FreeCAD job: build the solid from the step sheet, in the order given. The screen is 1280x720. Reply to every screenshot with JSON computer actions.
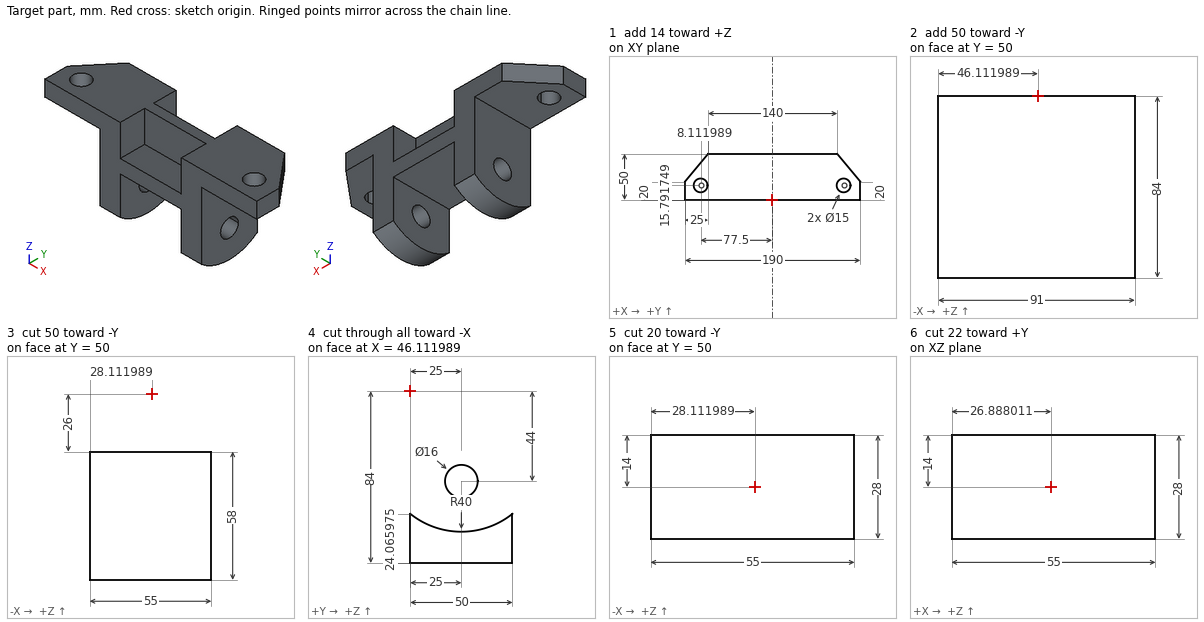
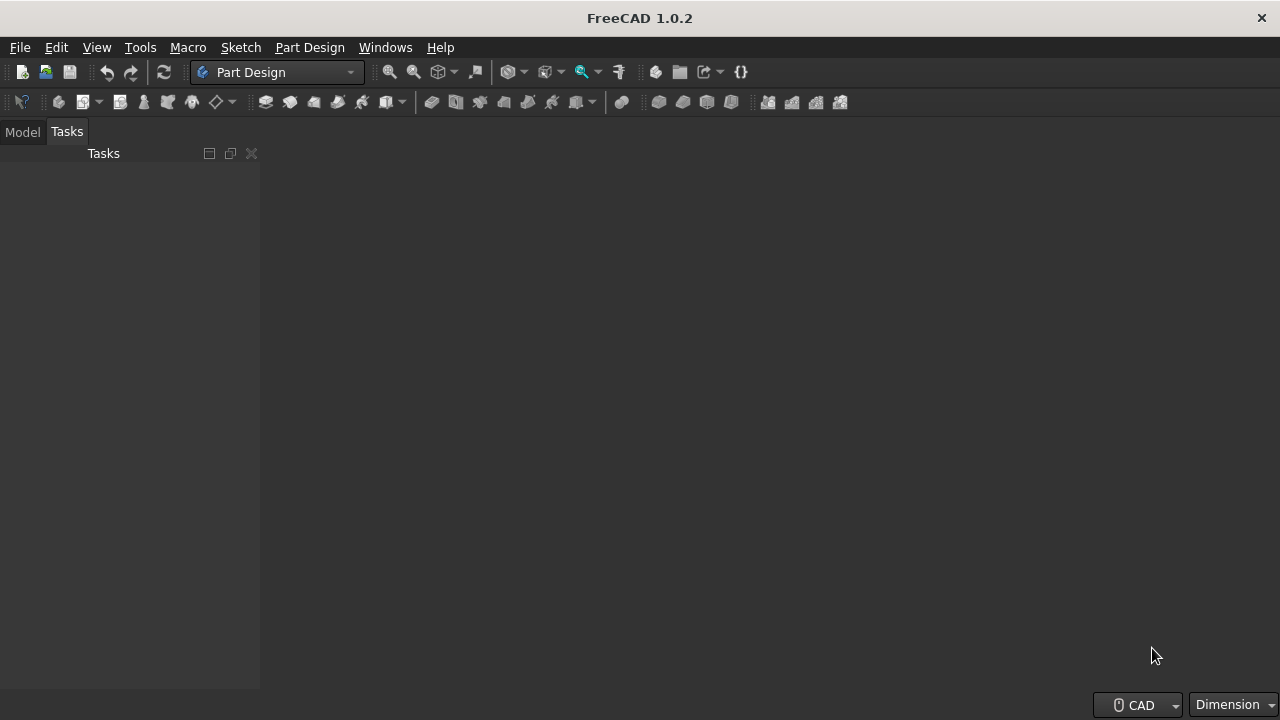
{"action": "left_click", "coordinate": [22, 72]}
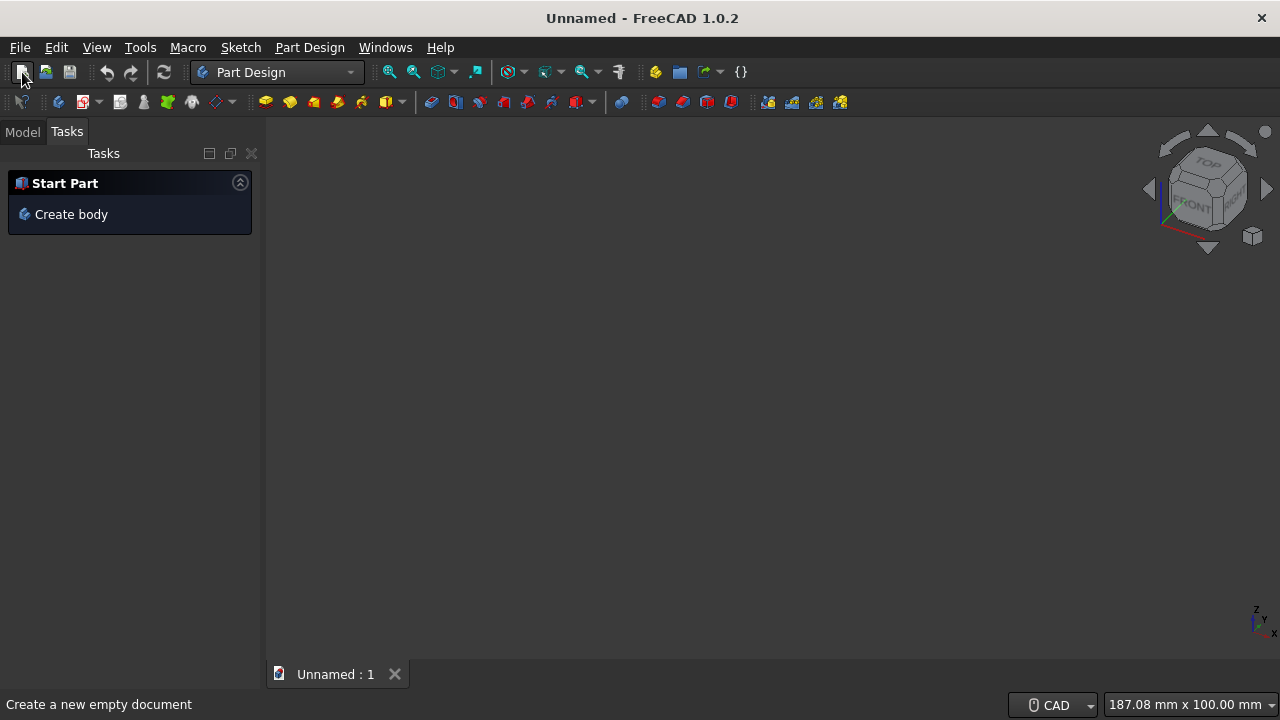
{"action": "left_click", "coordinate": [84, 102]}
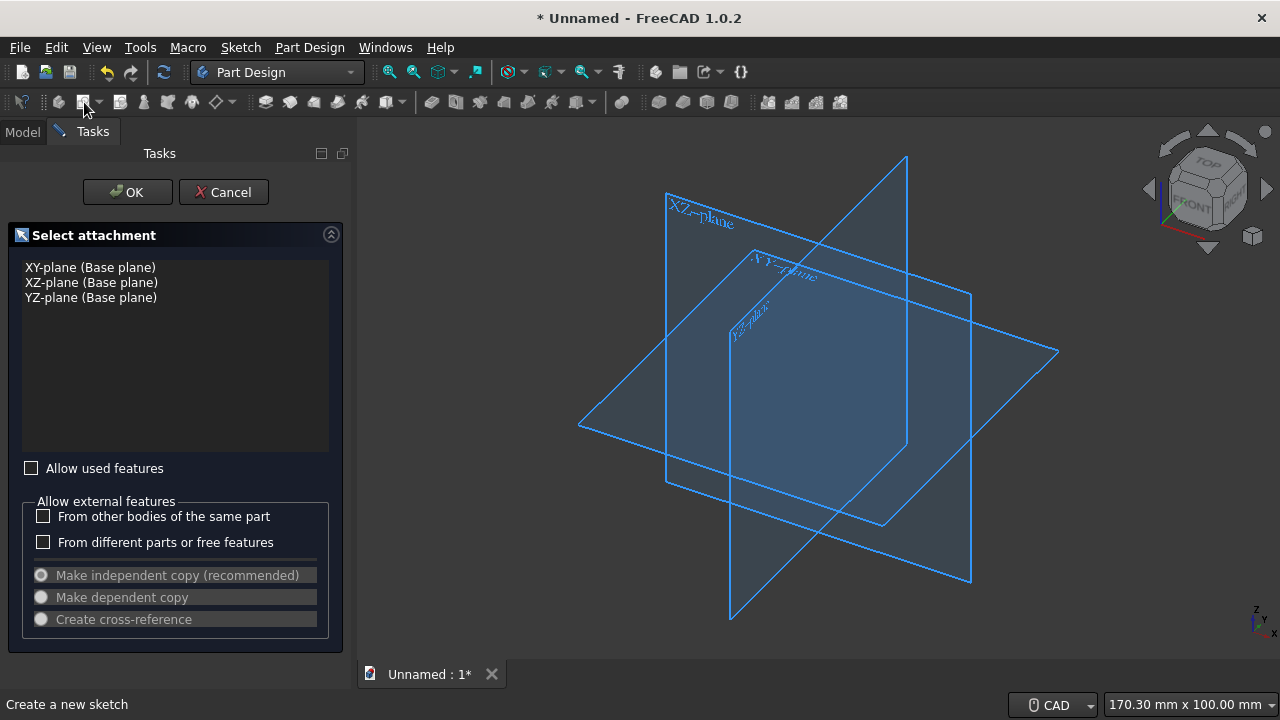
{"action": "left_click", "coordinate": [82, 268]}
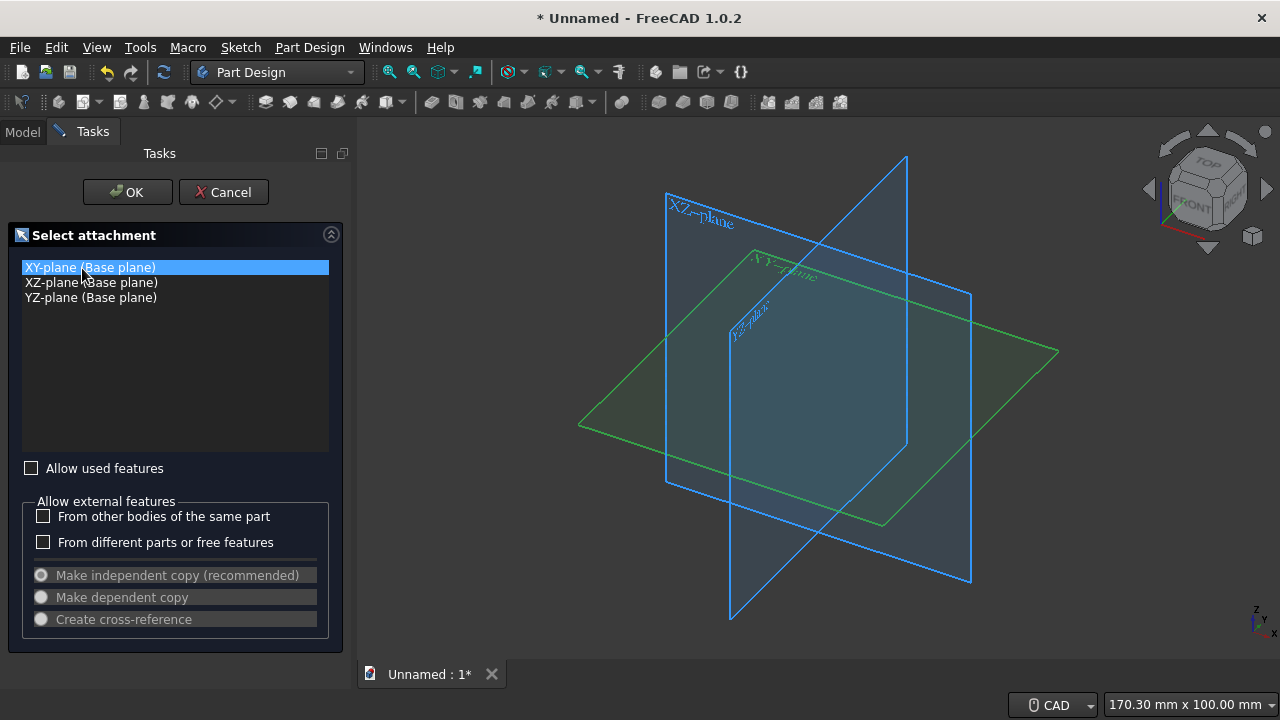
{"action": "left_click", "coordinate": [128, 192]}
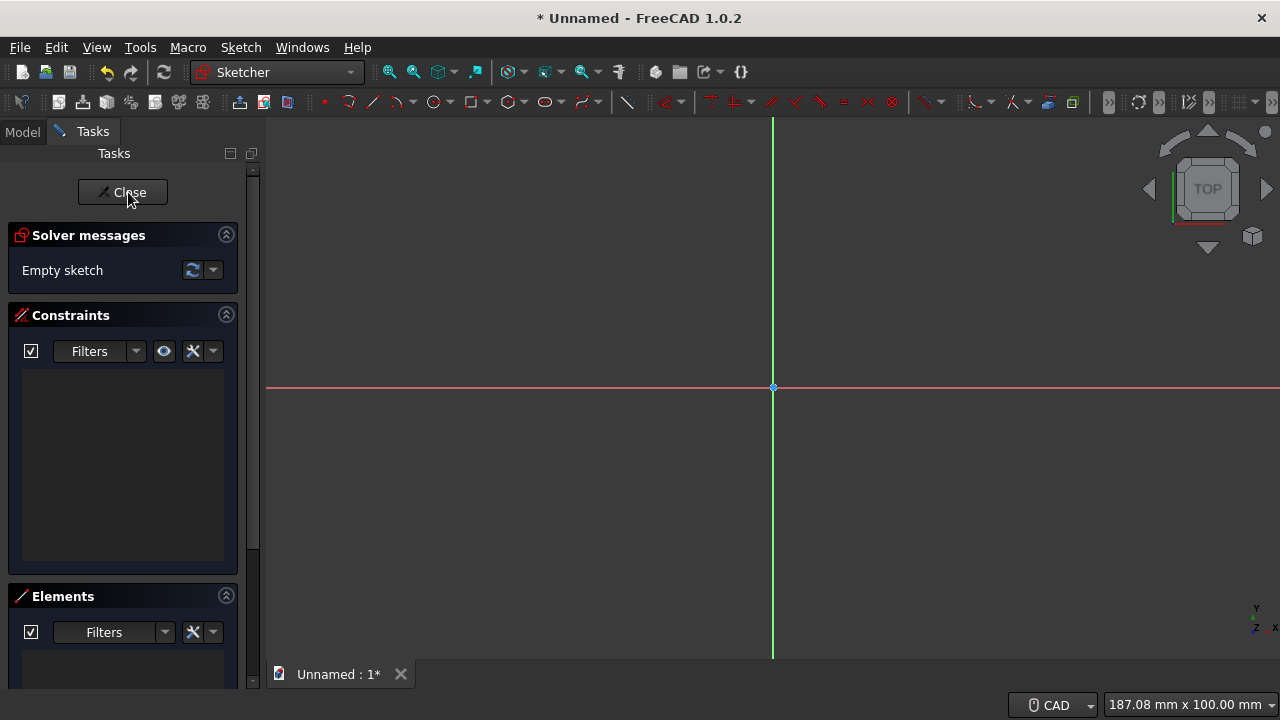
{"action": "scroll", "coordinate": [617, 553], "scroll_direction": "down", "scroll_amount": 3}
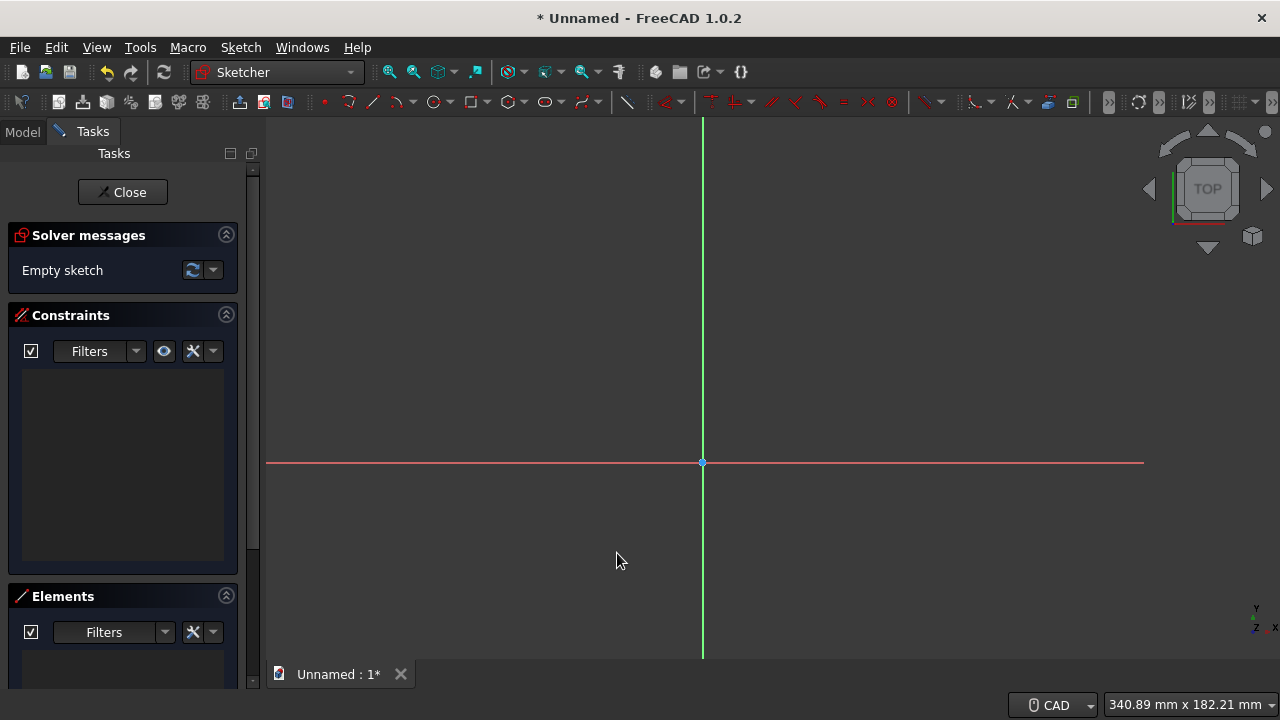
{"action": "left_click", "coordinate": [350, 102]}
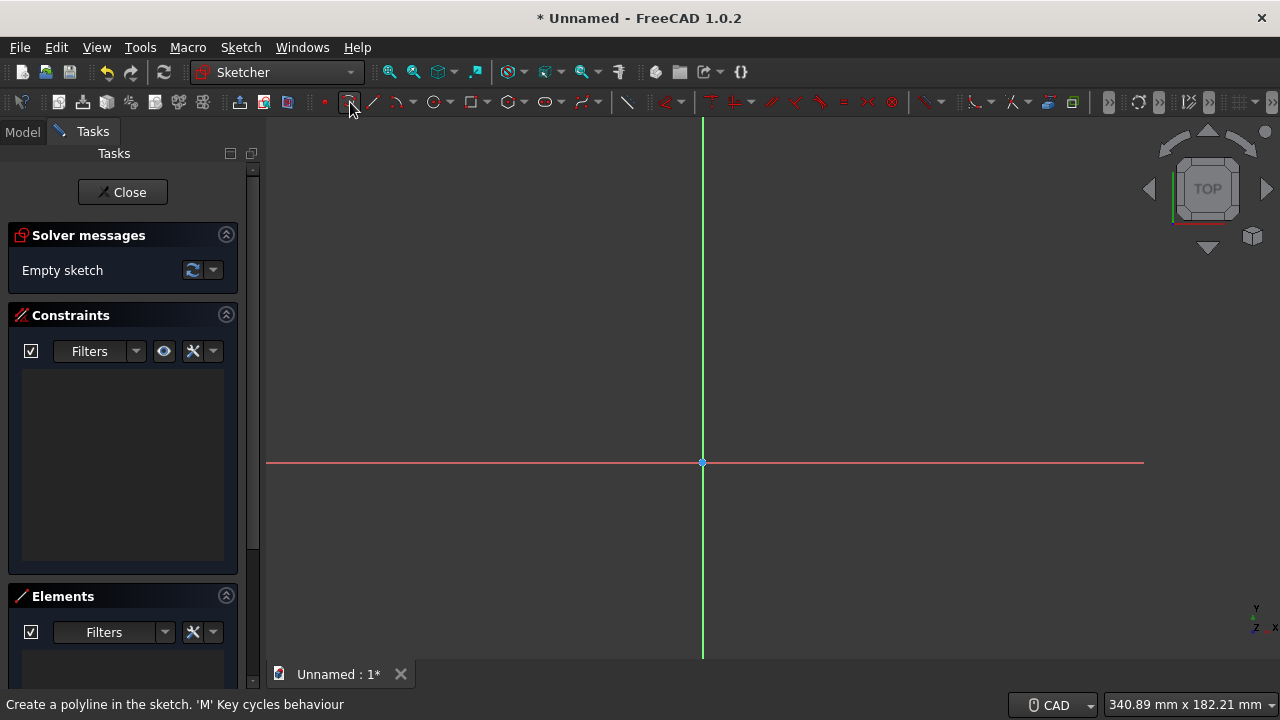
{"action": "left_click", "coordinate": [496, 314]}
{"action": "left_click", "coordinate": [422, 403]}
{"action": "left_click", "coordinate": [422, 463]}
{"action": "left_click", "coordinate": [987, 454]}
{"action": "left_click", "coordinate": [987, 403]}
{"action": "left_click", "coordinate": [913, 314]}
{"action": "left_click", "coordinate": [496, 315]}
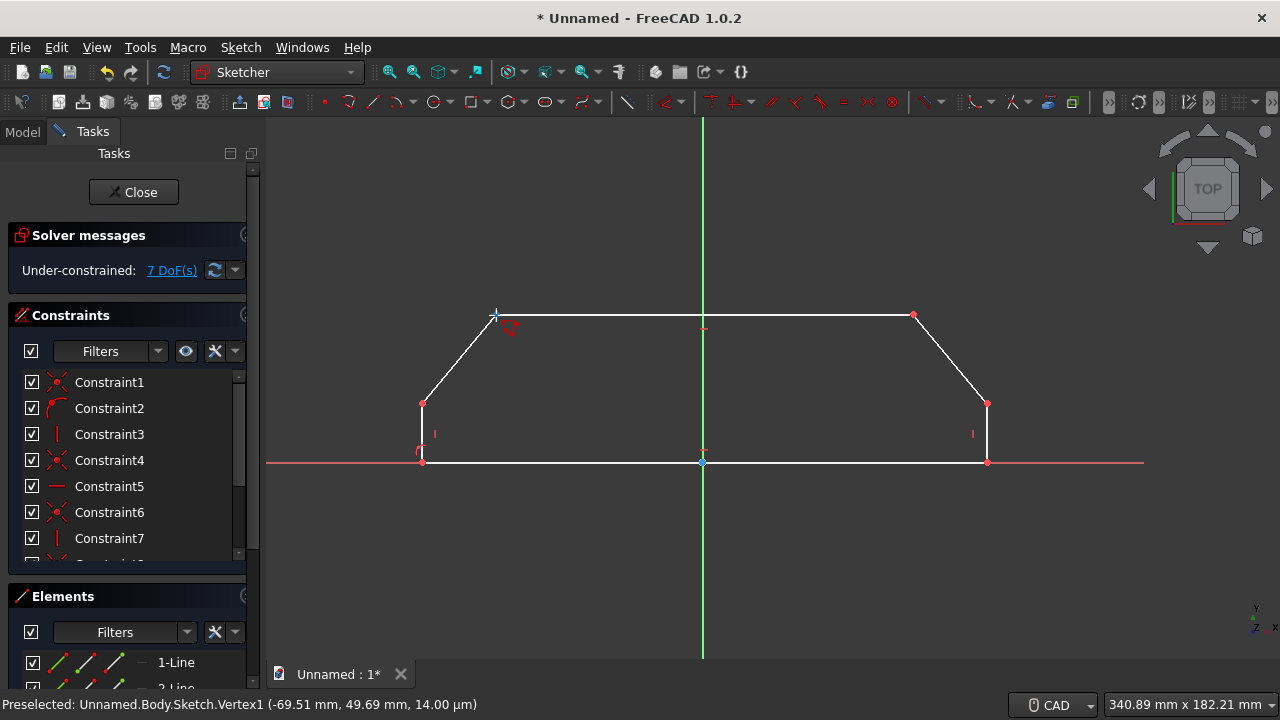
{"action": "left_click", "coordinate": [434, 102]}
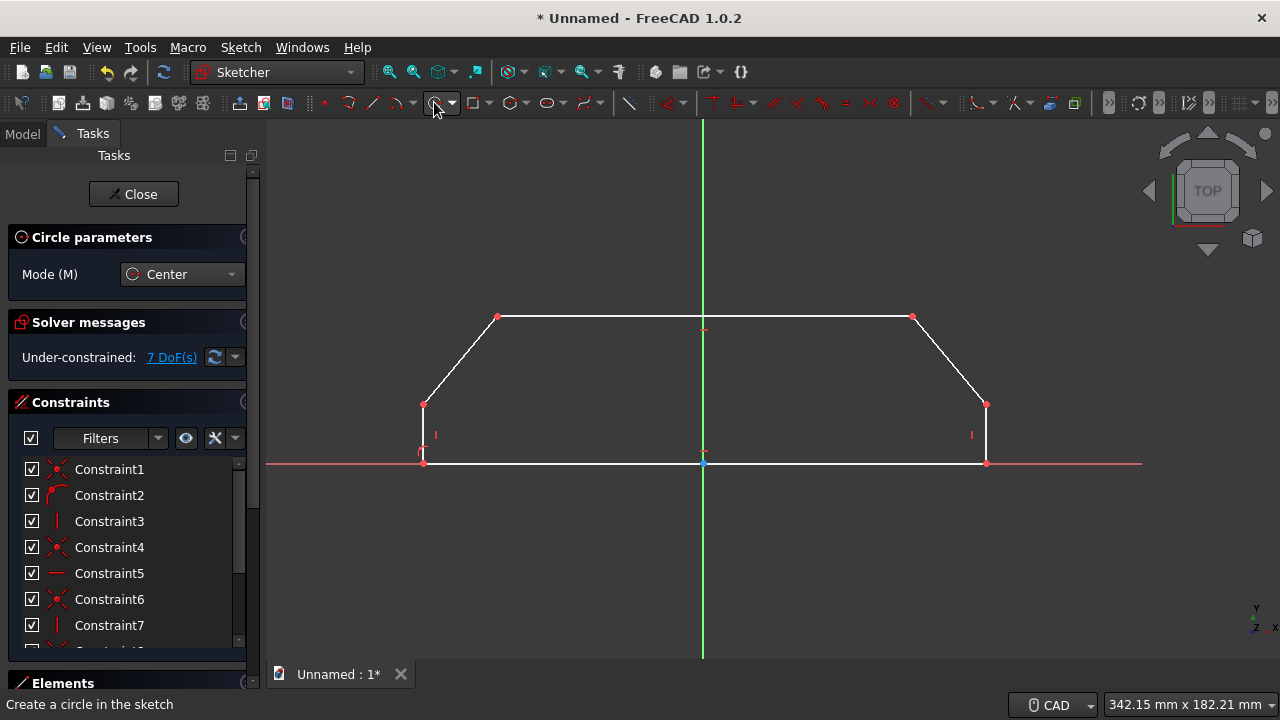
{"action": "left_click", "coordinate": [473, 417]}
{"action": "mouse_move", "coordinate": [489, 401]}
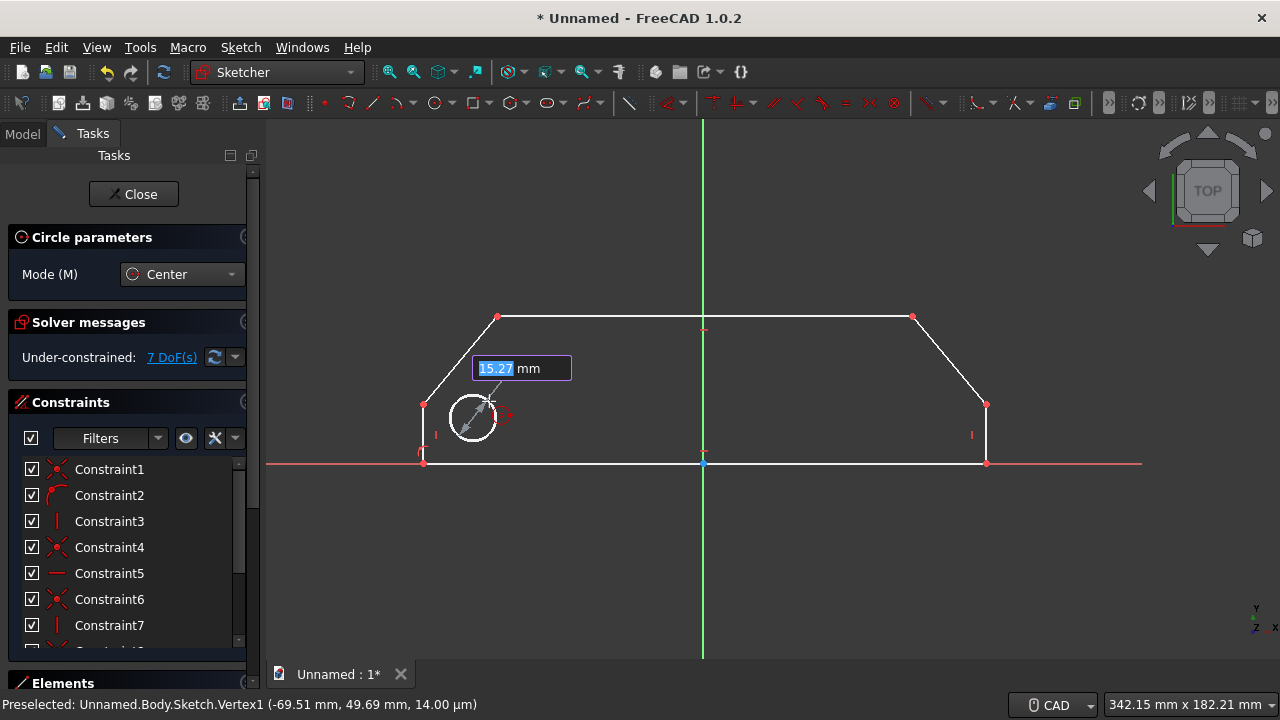
{"action": "type", "text": "15"}
{"action": "key", "text": "Return"}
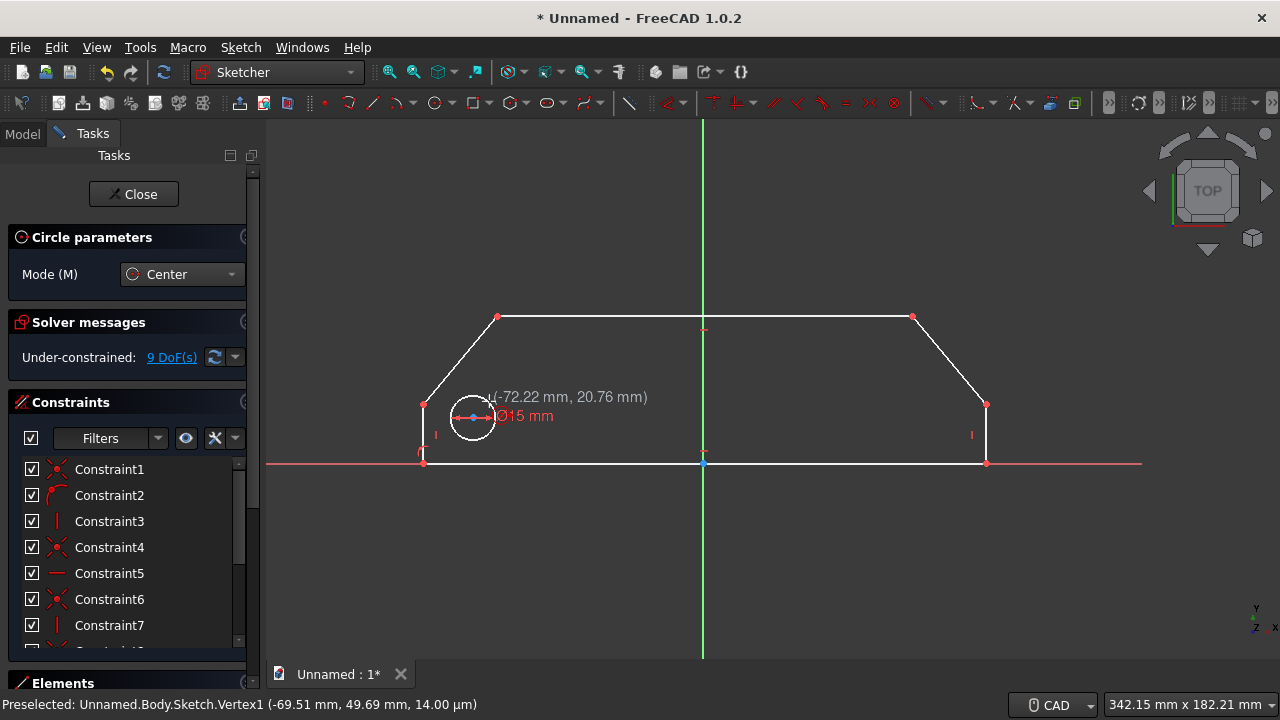
{"action": "left_click", "coordinate": [933, 417]}
{"action": "mouse_move", "coordinate": [948, 401]}